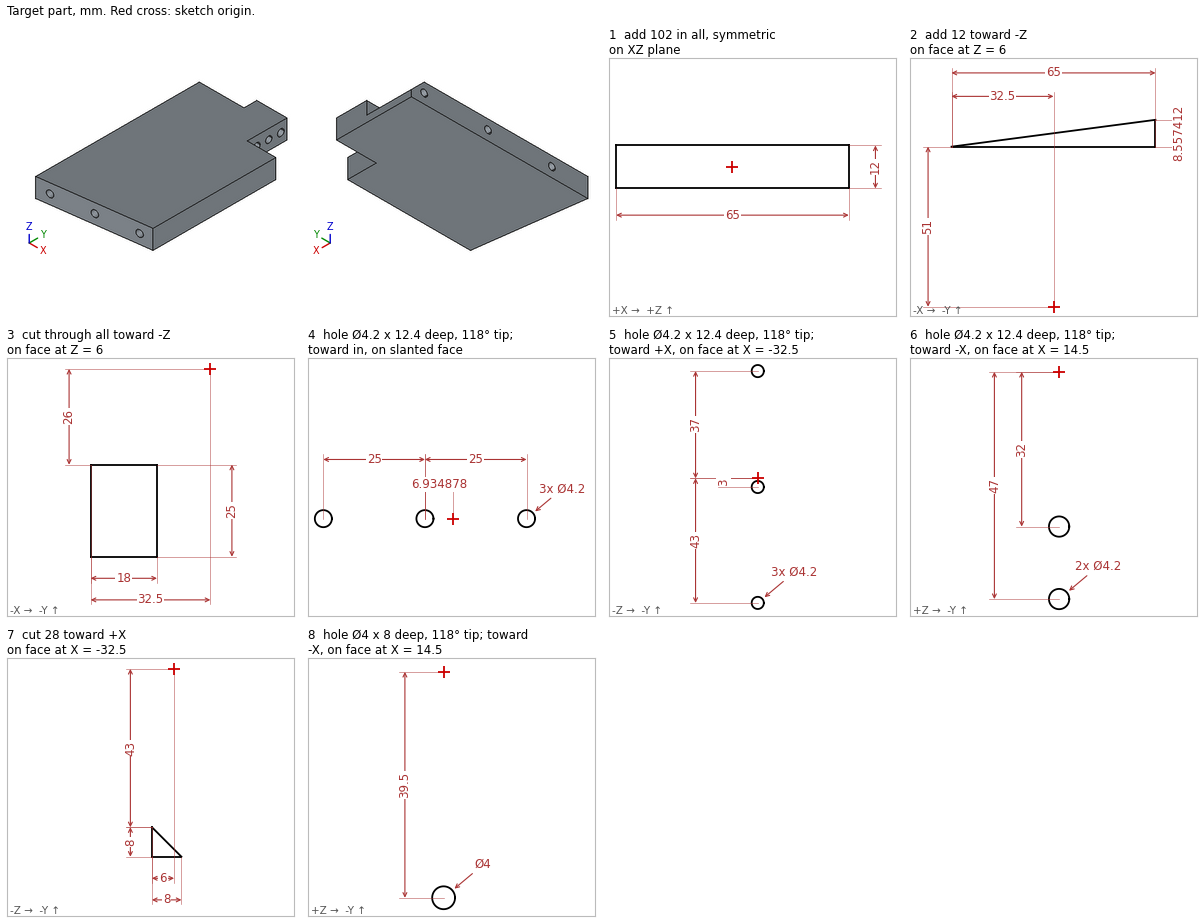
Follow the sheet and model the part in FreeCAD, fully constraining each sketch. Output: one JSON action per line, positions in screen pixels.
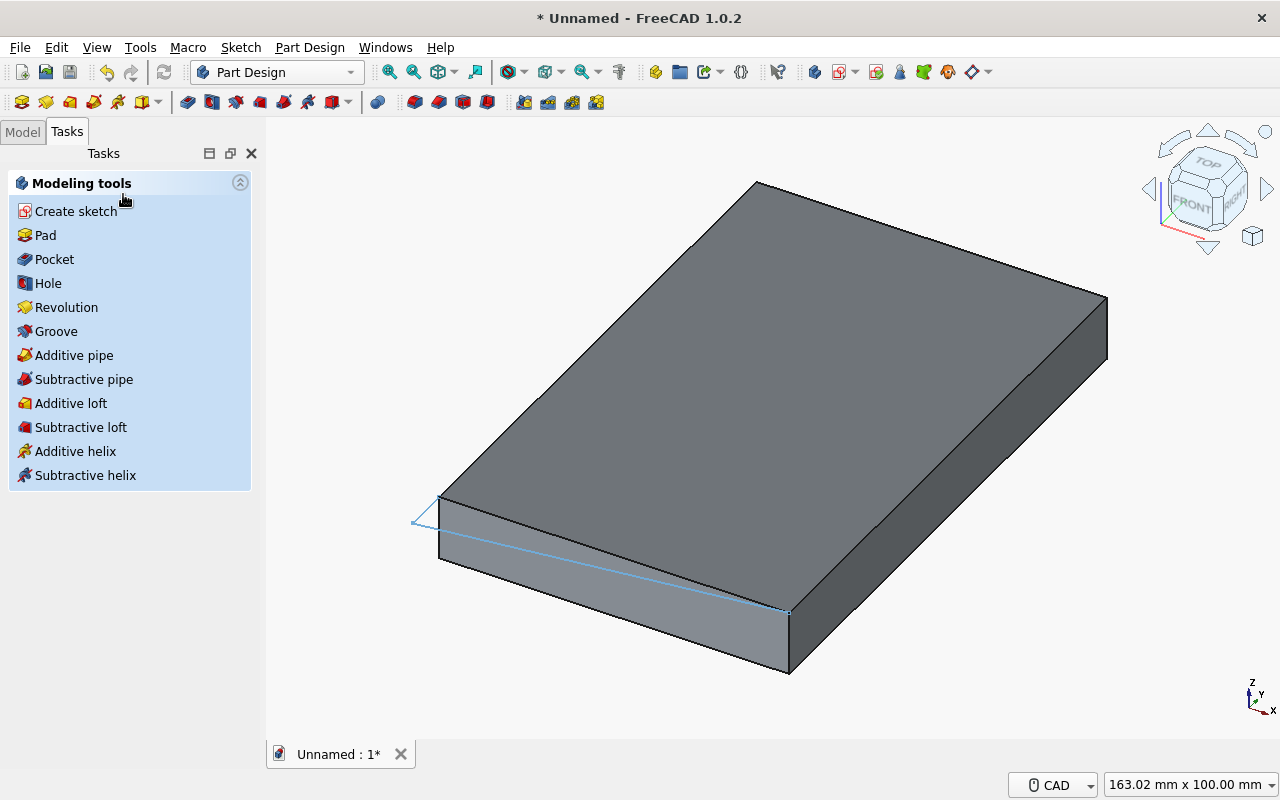
{"action": "left_click", "coordinate": [22, 102]}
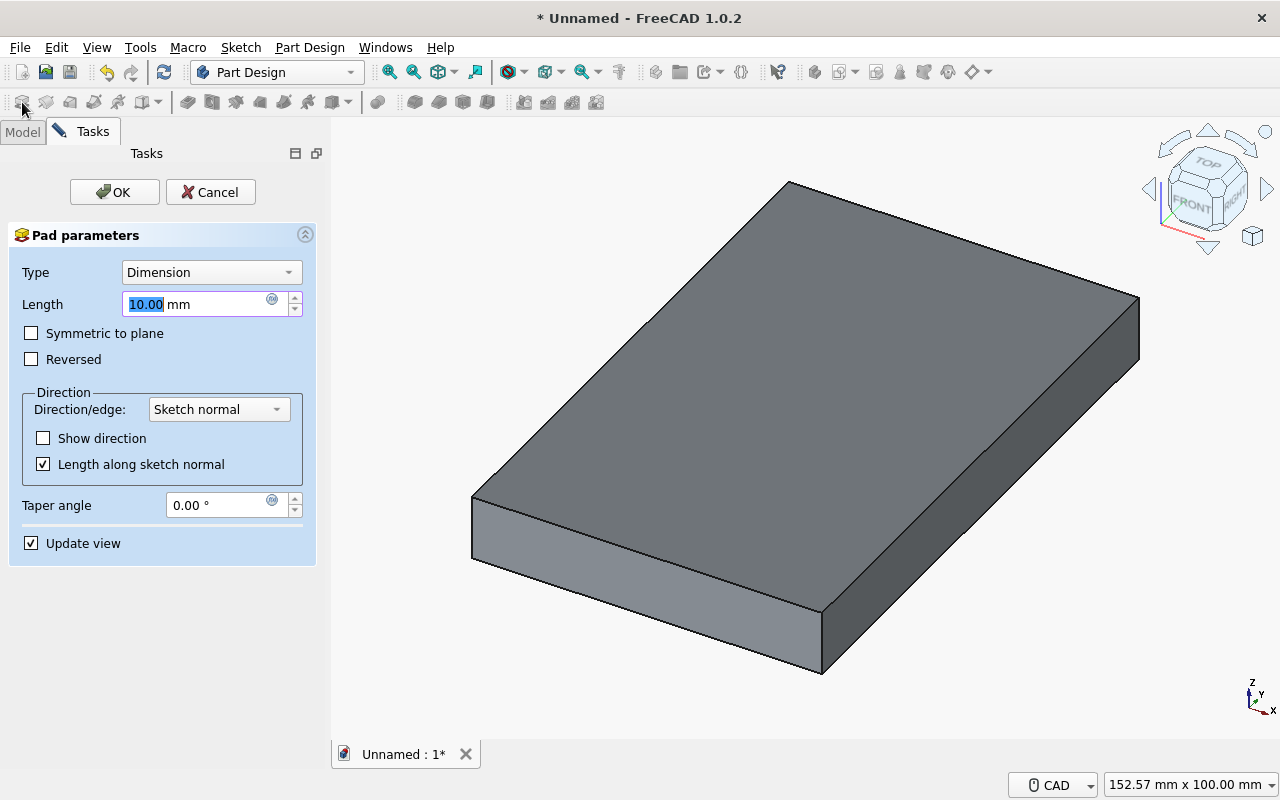
{"action": "type", "text": "12"}
{"action": "key", "text": "Tab"}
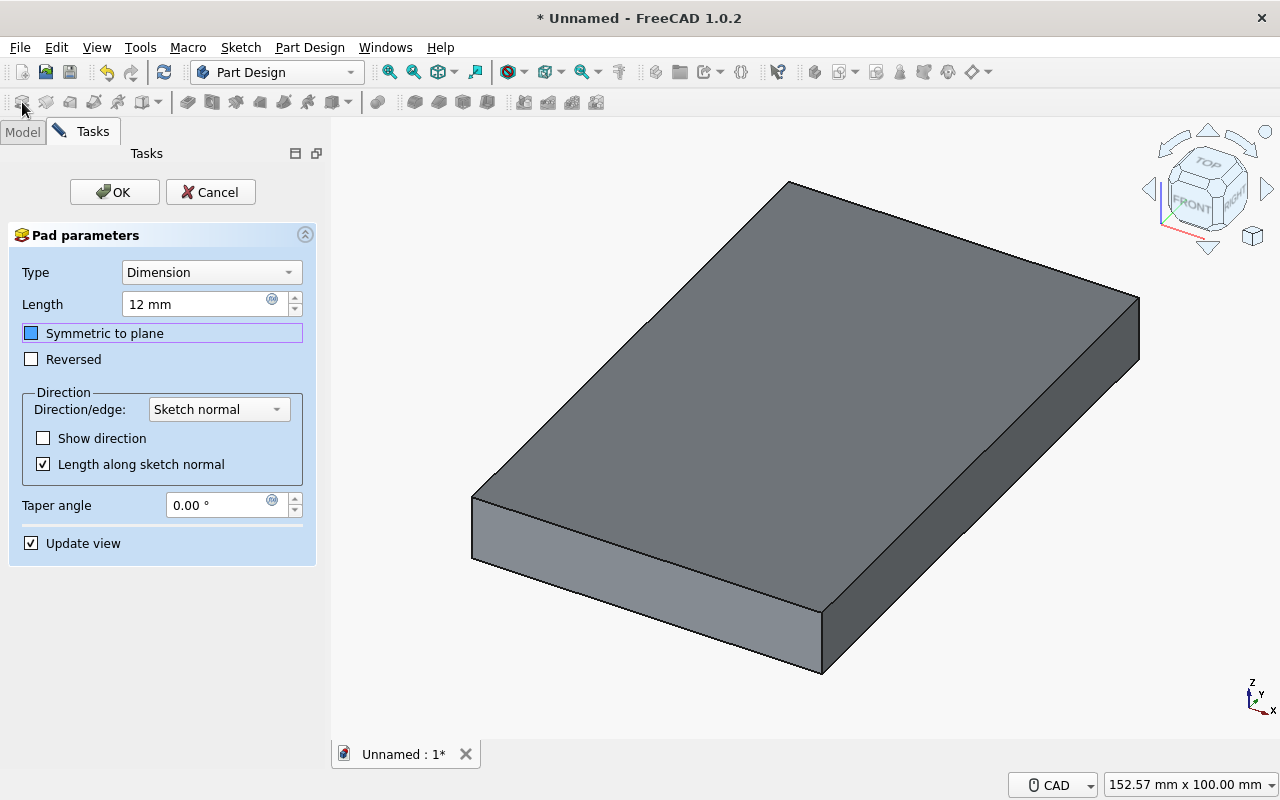
{"action": "left_click", "coordinate": [30, 359]}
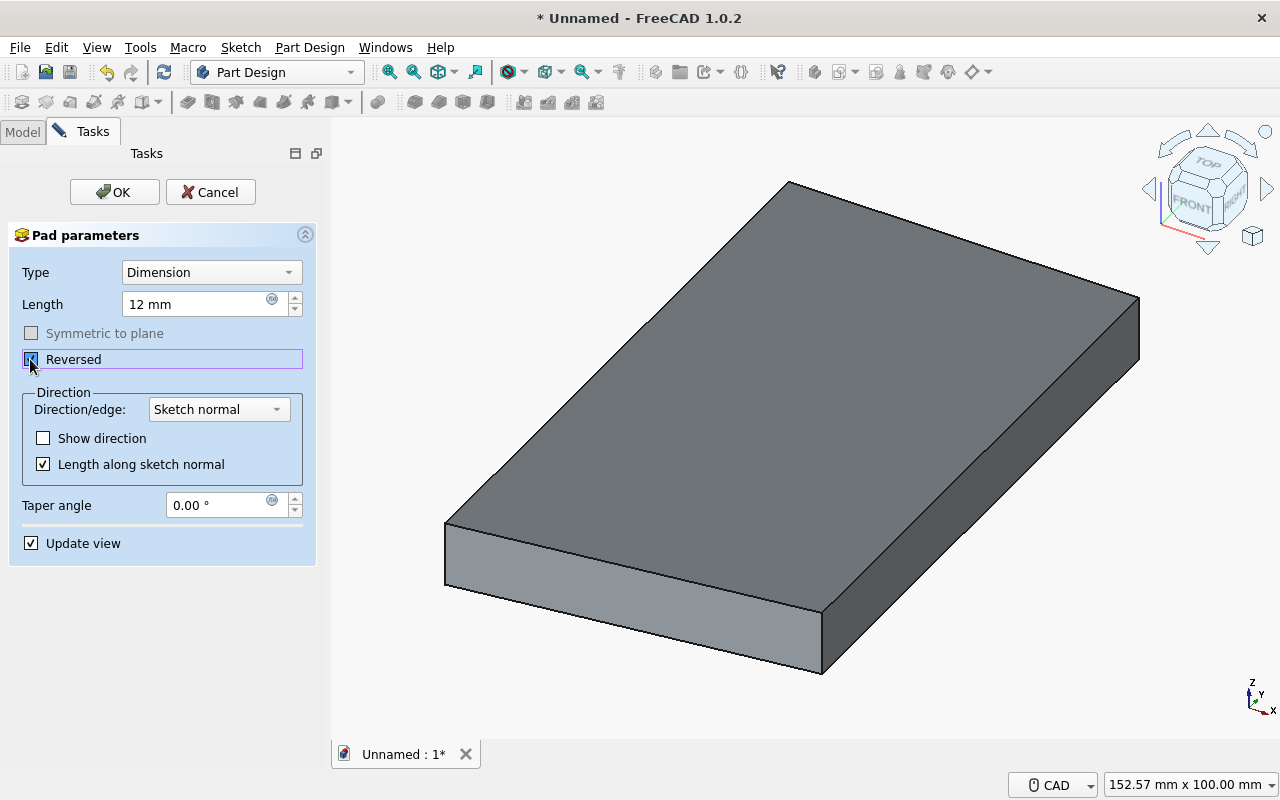
{"action": "left_click", "coordinate": [115, 192]}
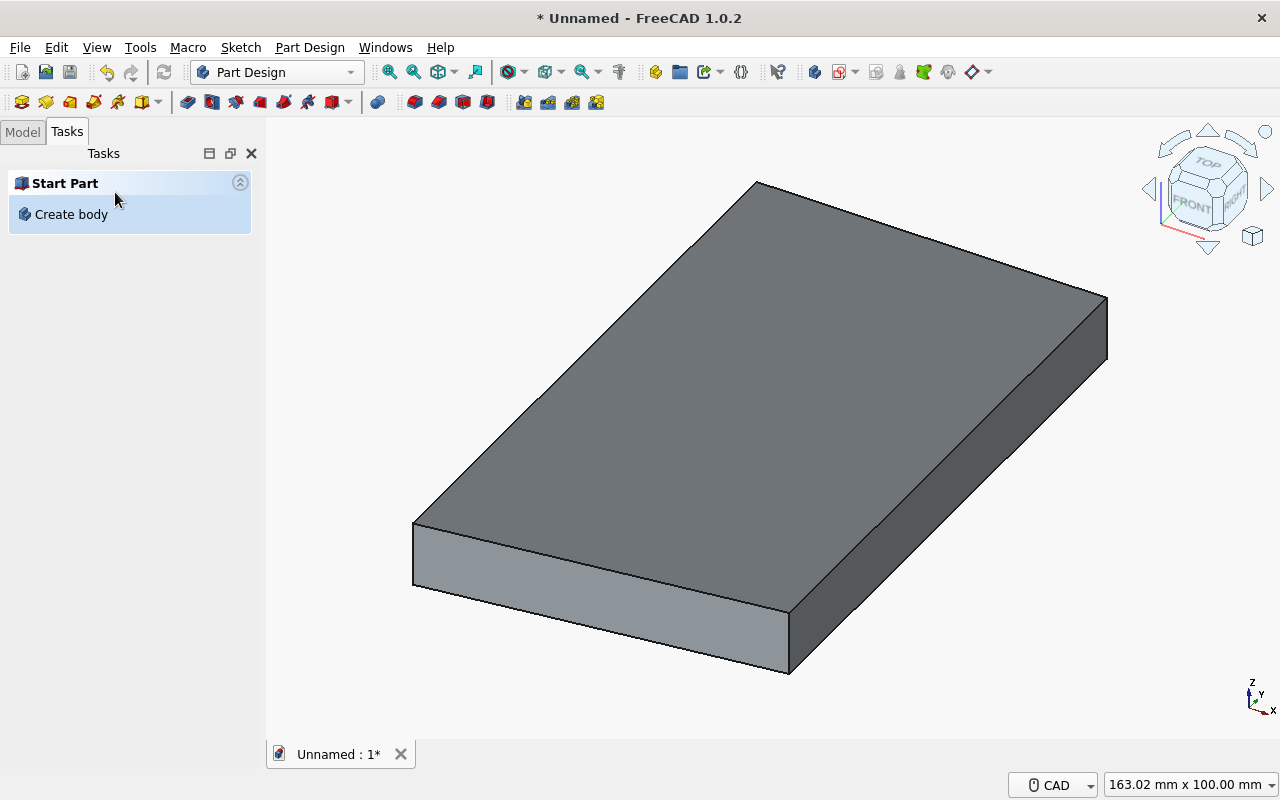
{"action": "left_click", "coordinate": [809, 361]}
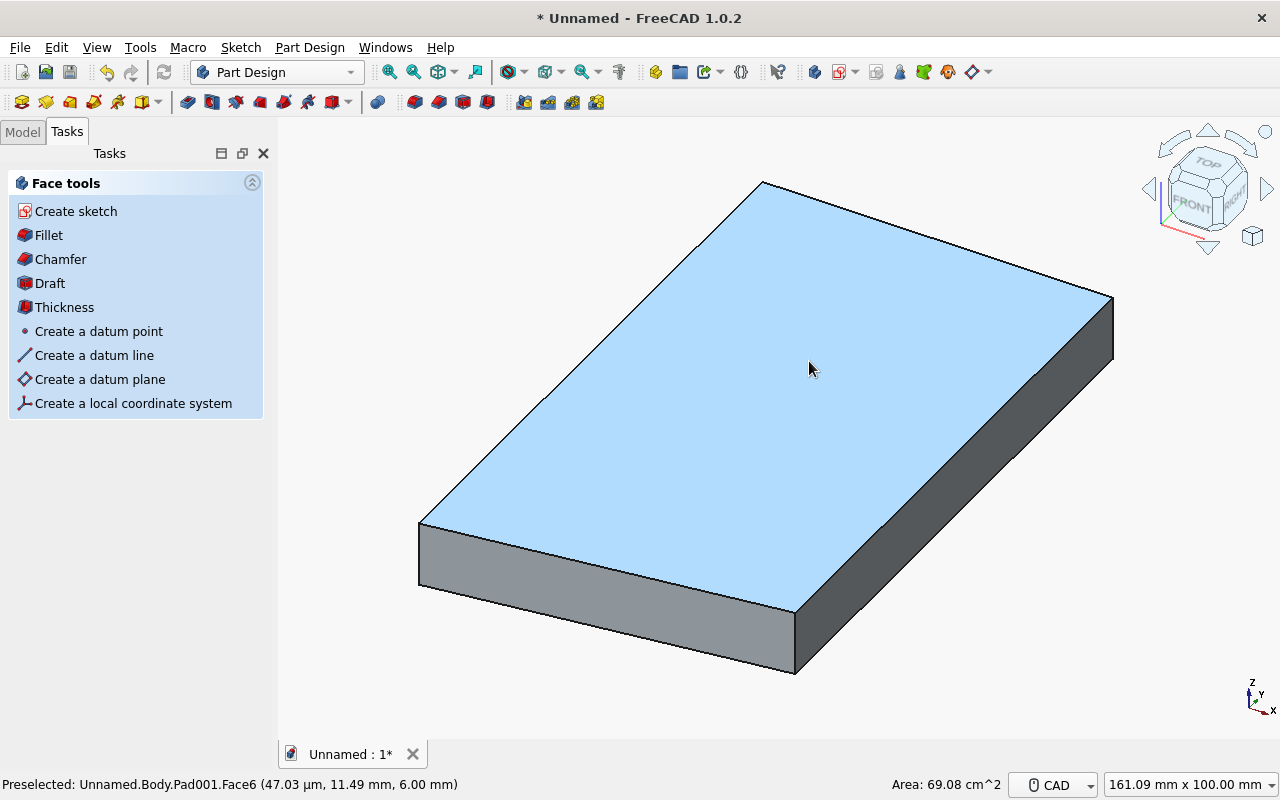
{"action": "left_click", "coordinate": [840, 72]}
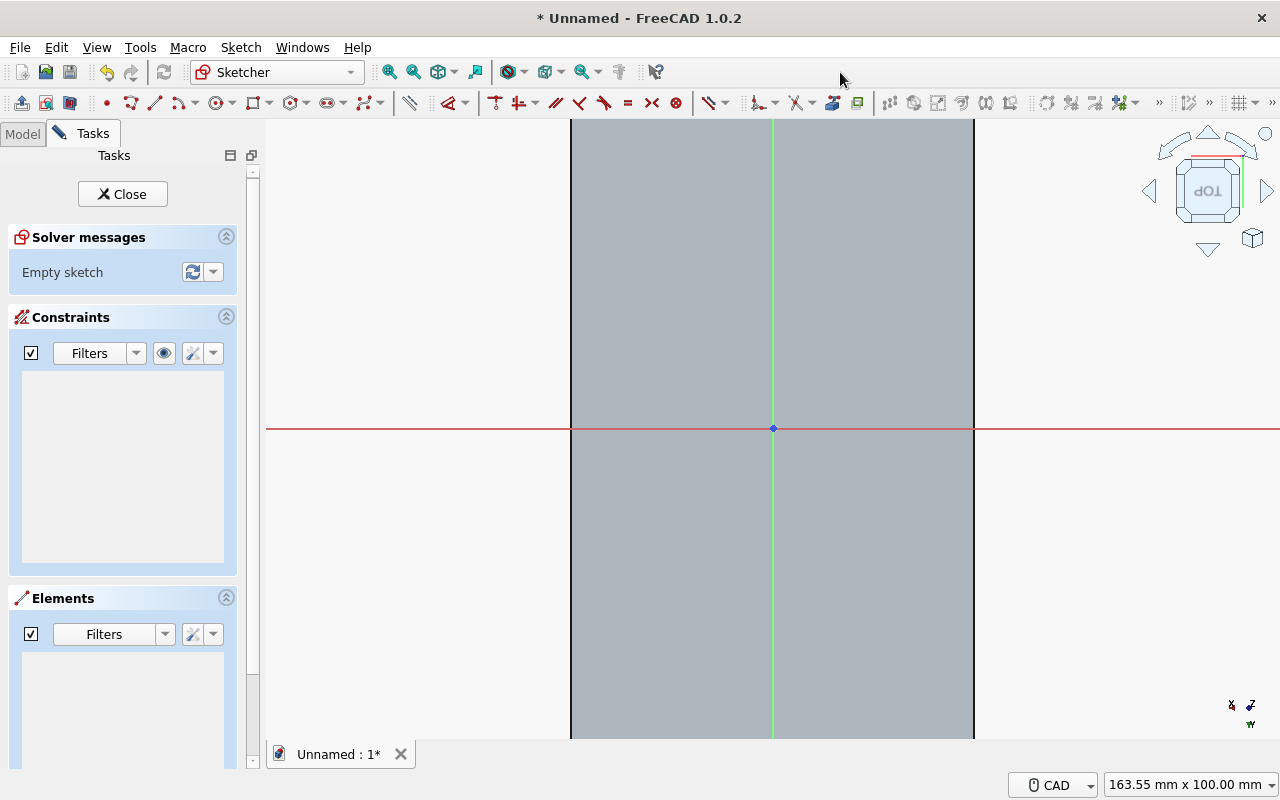
{"action": "scroll", "coordinate": [850, 147], "scroll_direction": "down", "scroll_amount": 1}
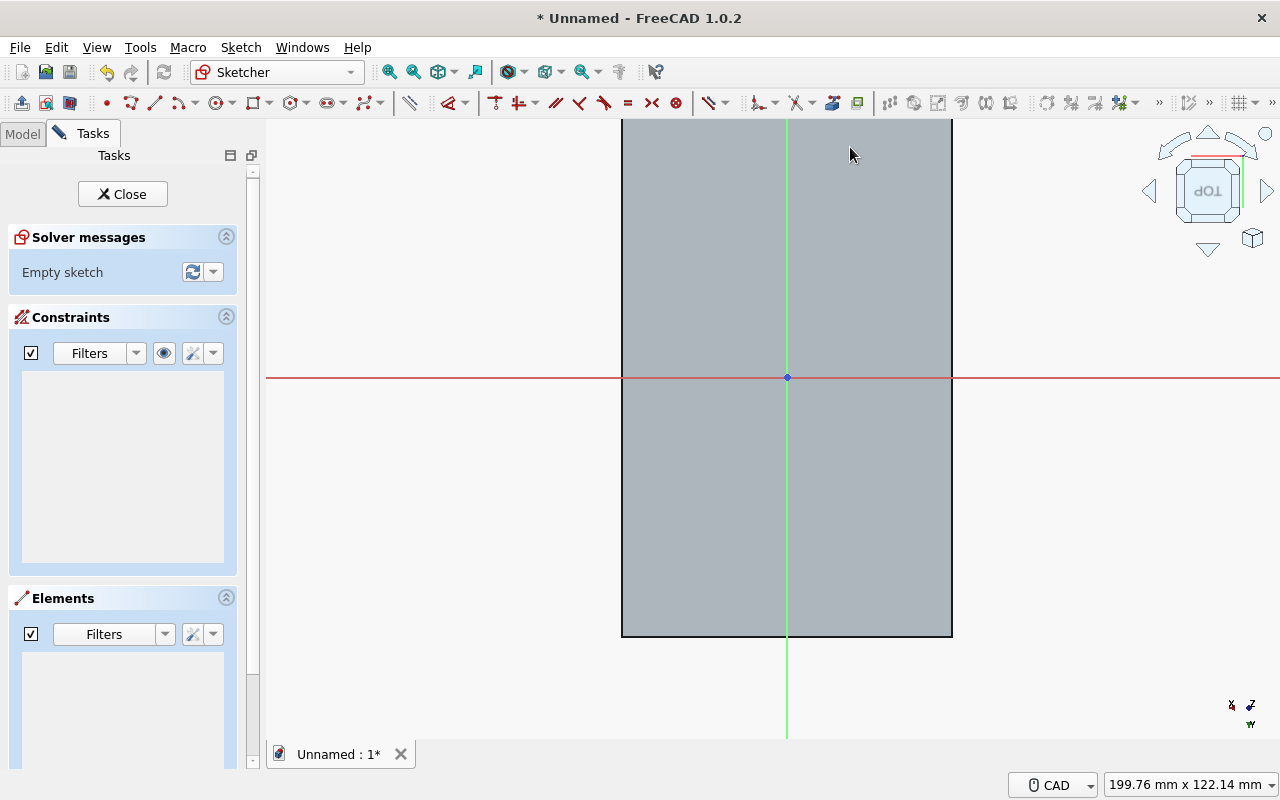
{"action": "scroll", "coordinate": [705, 667], "scroll_direction": "up", "scroll_amount": 2}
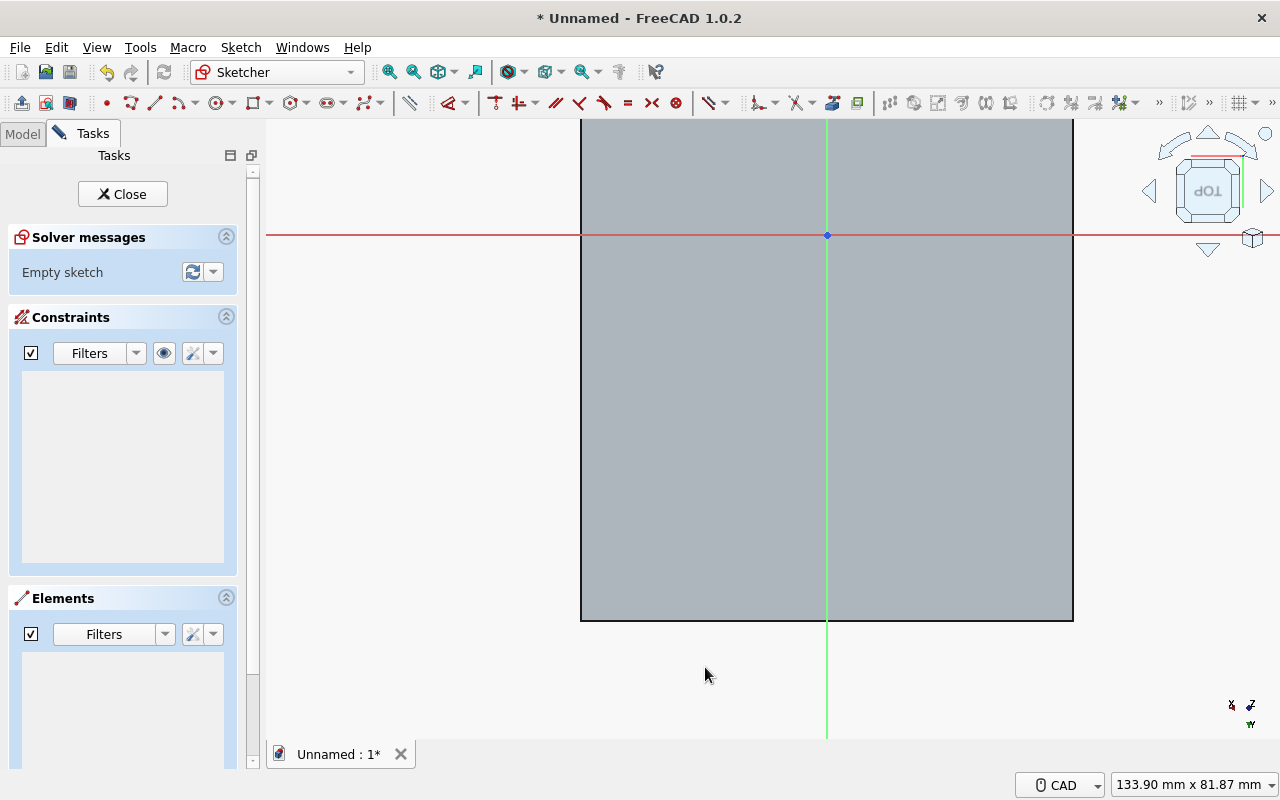
{"action": "key", "text": "g r"}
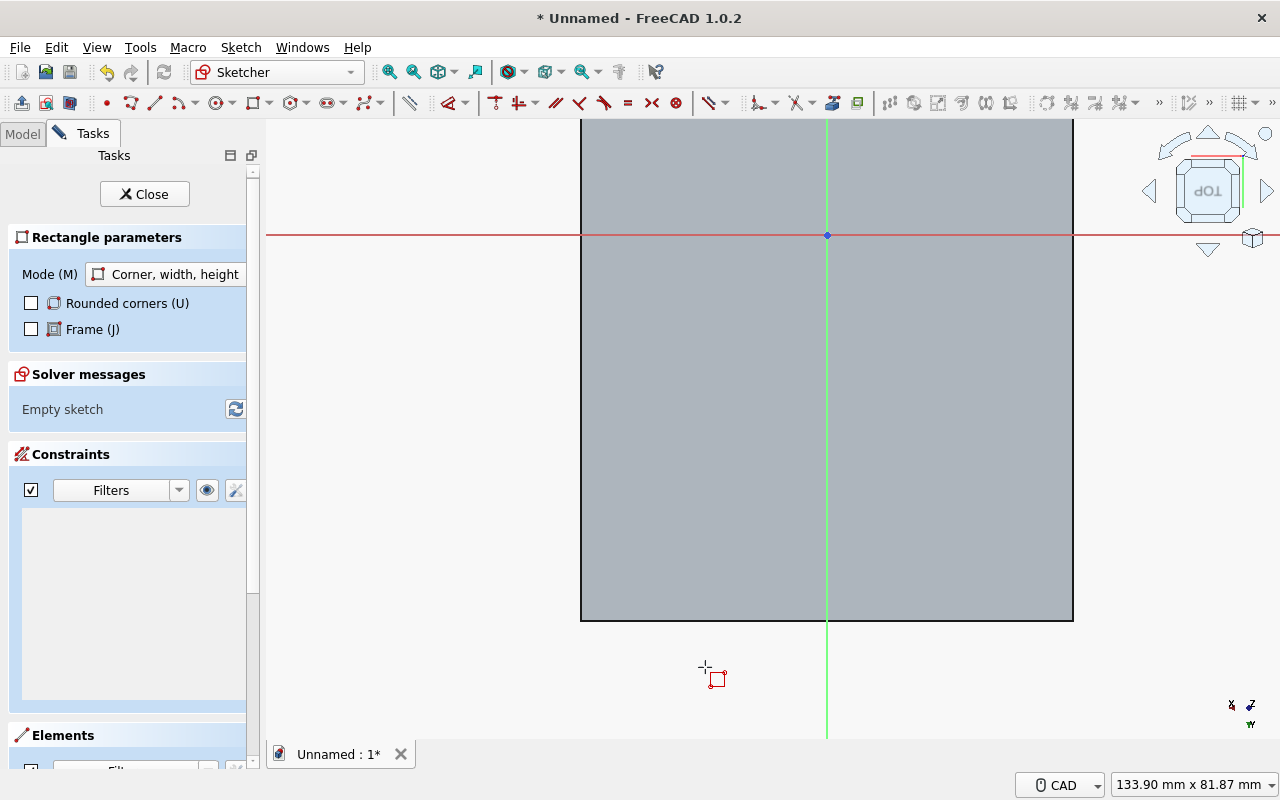
{"action": "left_click", "coordinate": [581, 432]}
{"action": "mouse_move", "coordinate": [717, 621]}